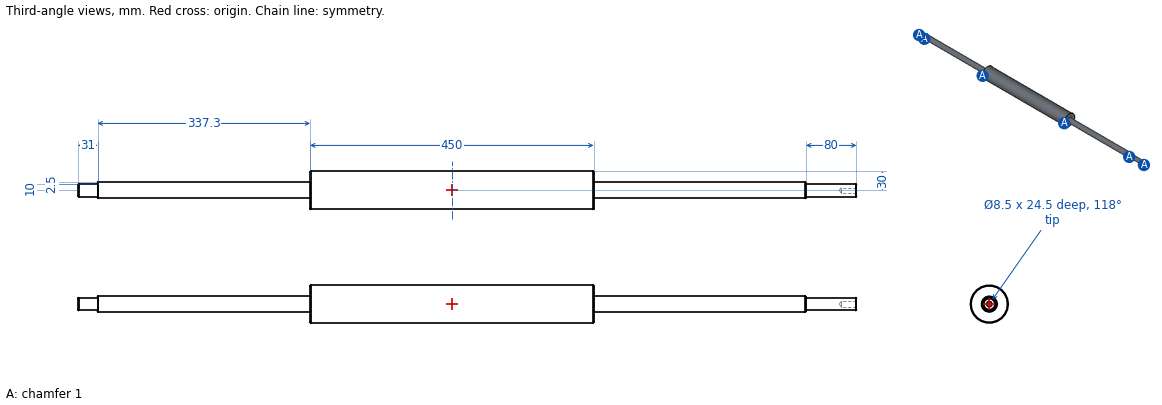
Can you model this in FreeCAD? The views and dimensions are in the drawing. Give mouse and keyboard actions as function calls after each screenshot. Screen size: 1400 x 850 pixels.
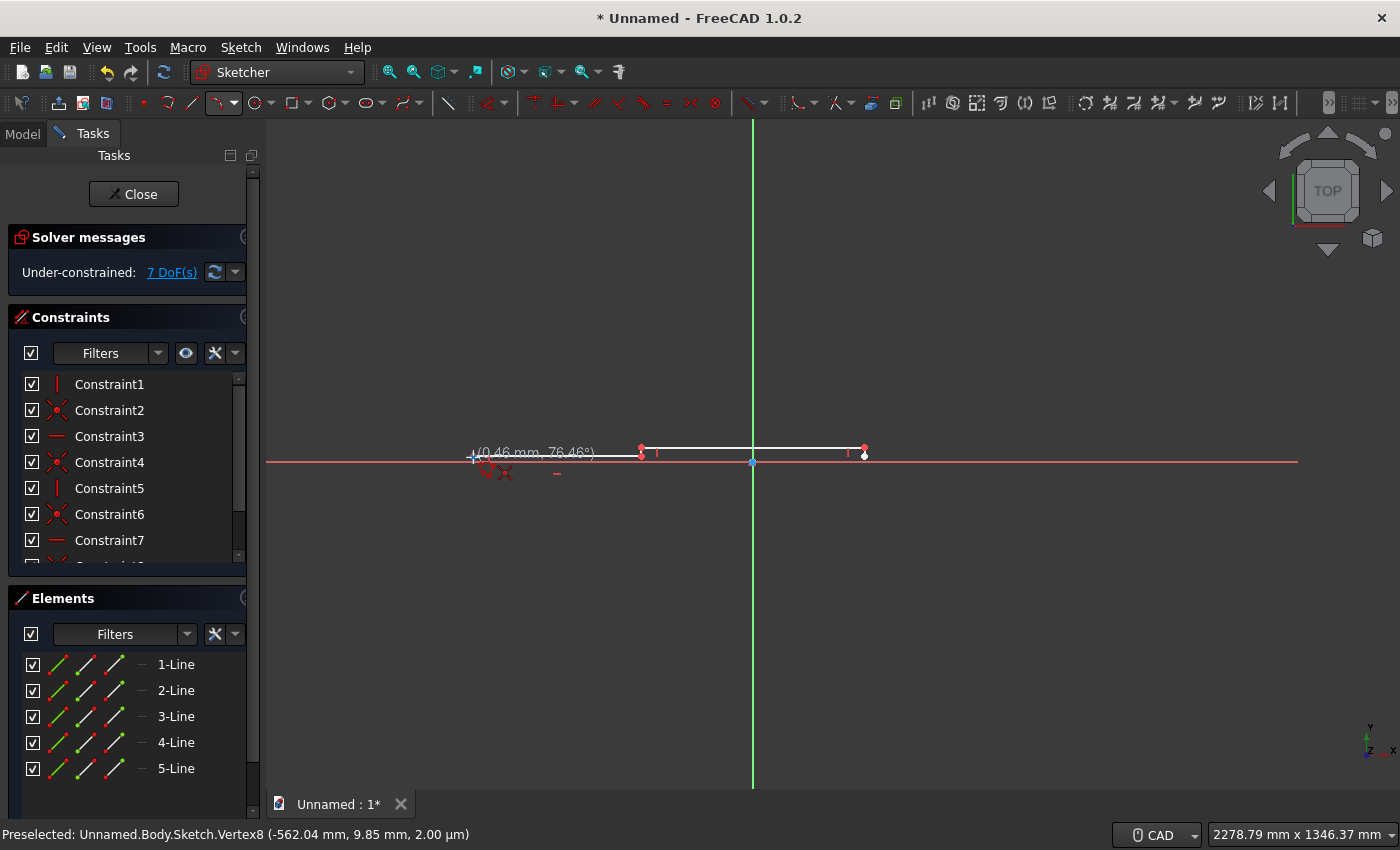
scroll(458, 457, up, 6)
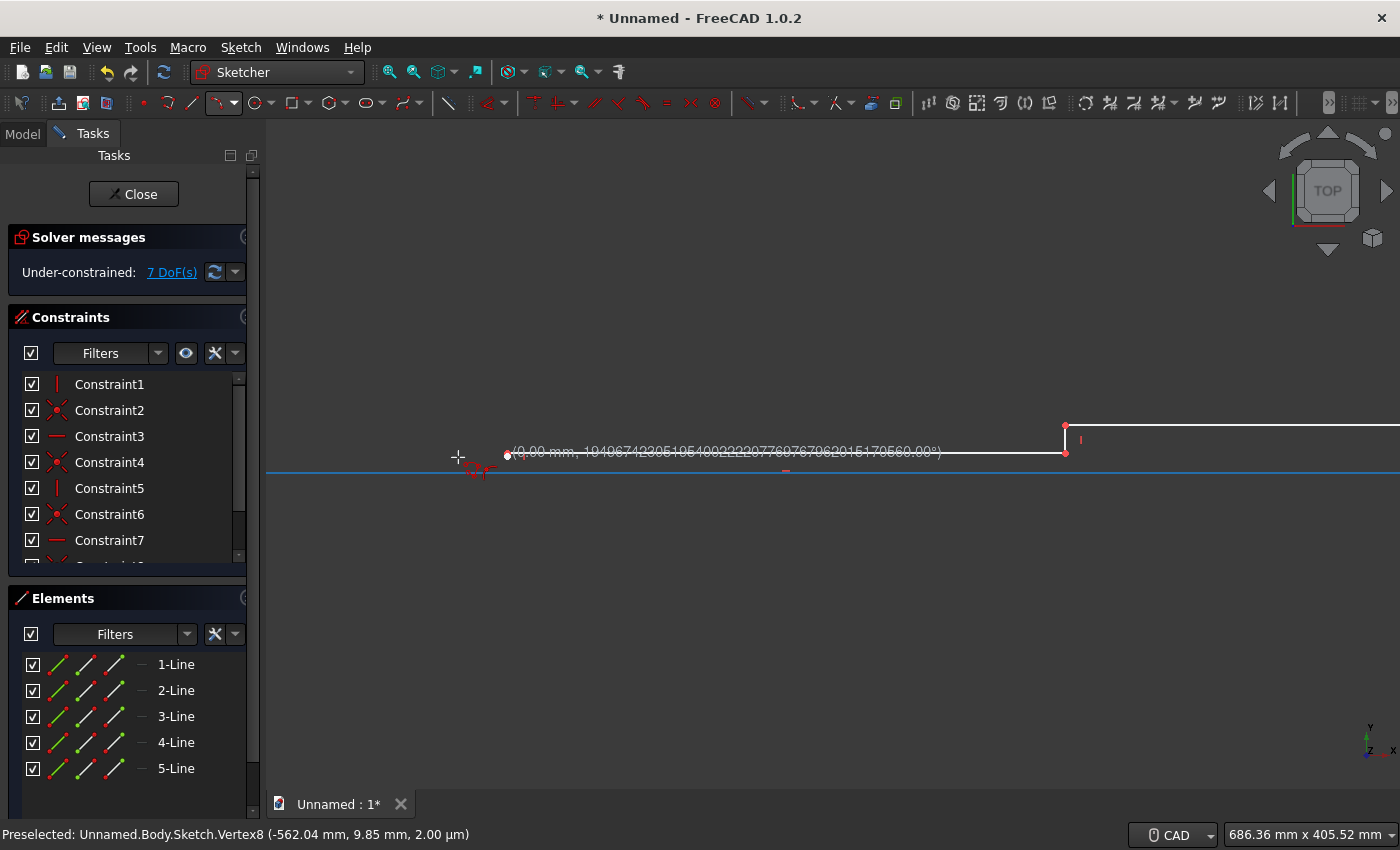
click(456, 457)
click(456, 473)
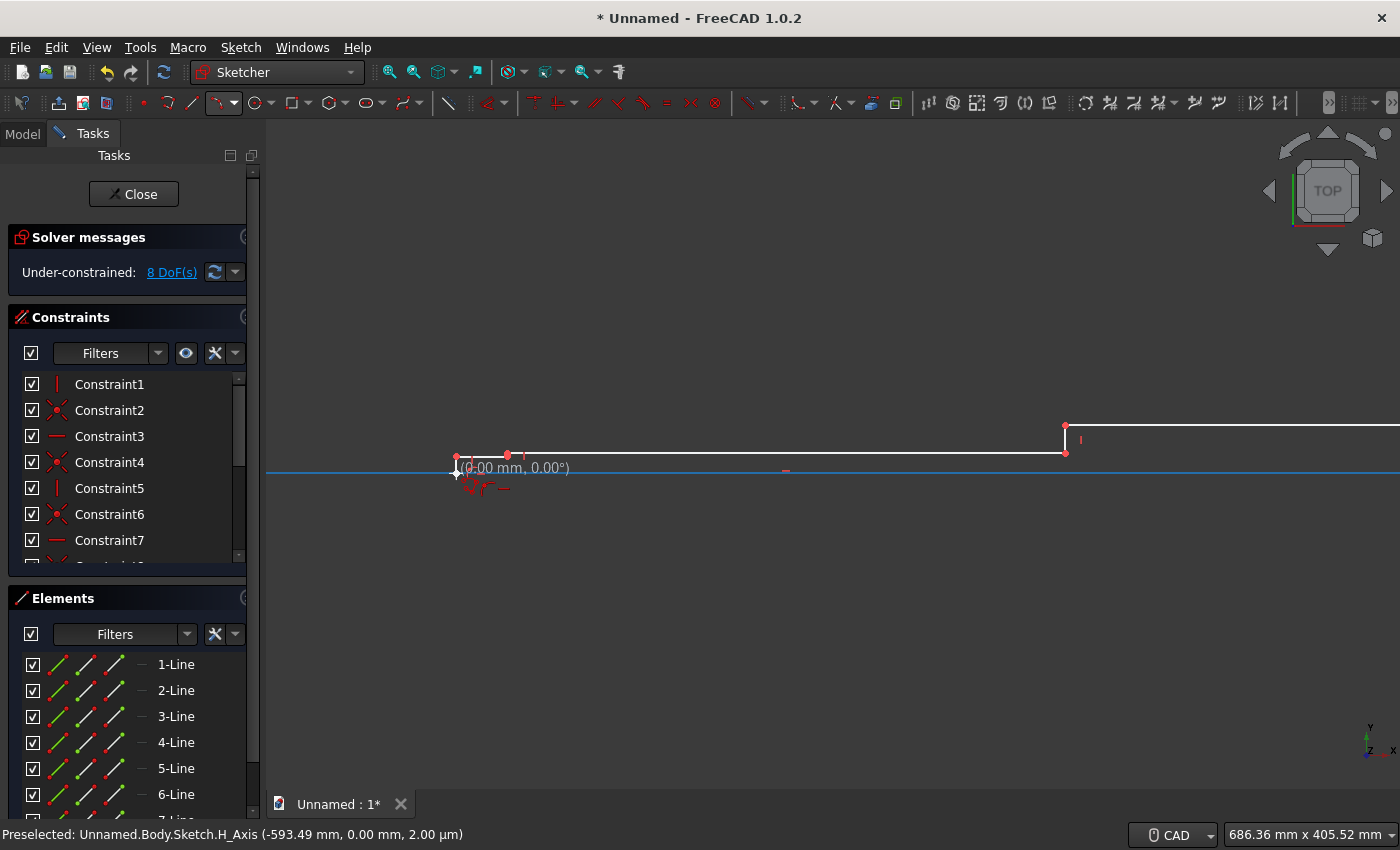
scroll(457, 456, down, 6)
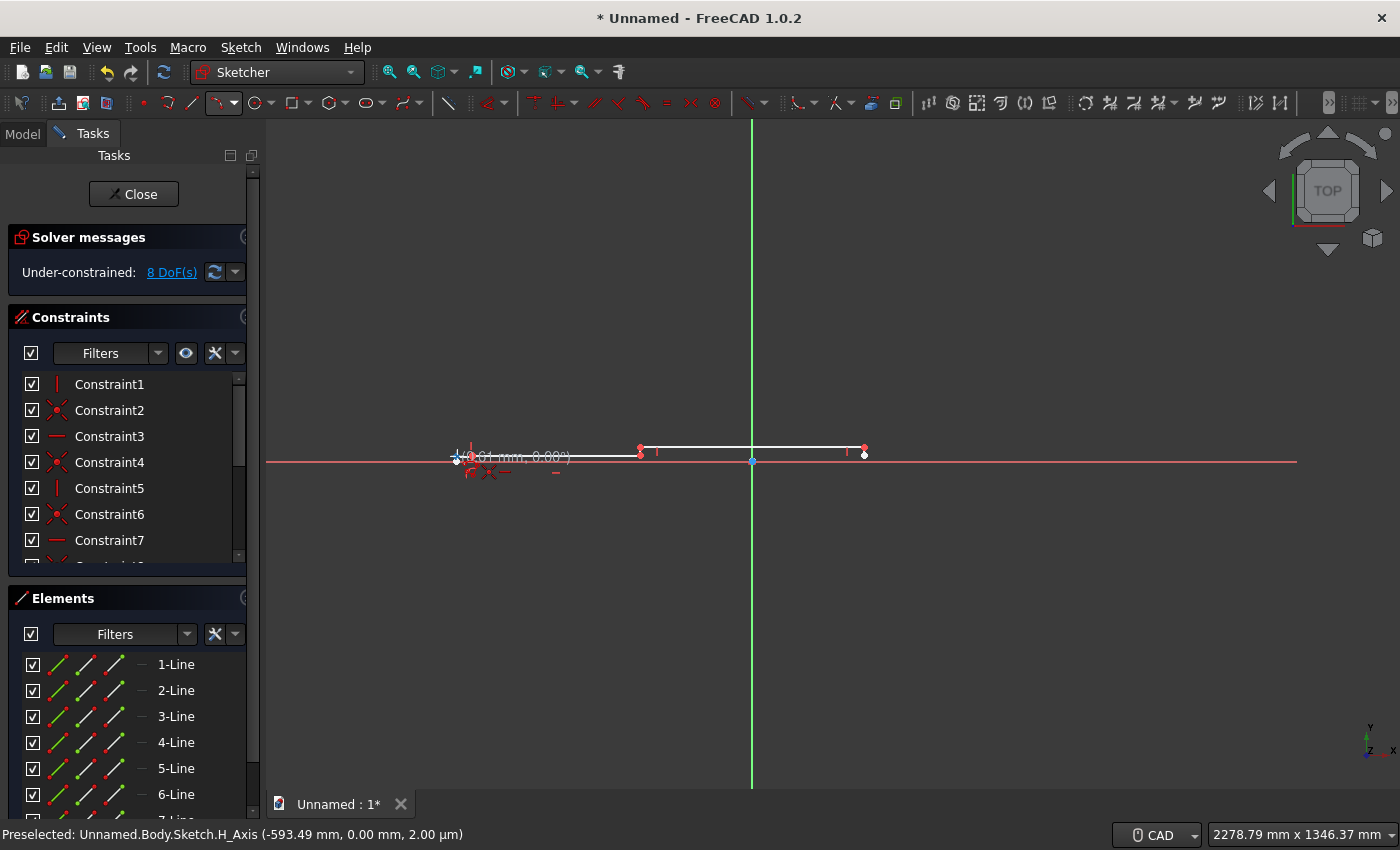
click(1072, 453)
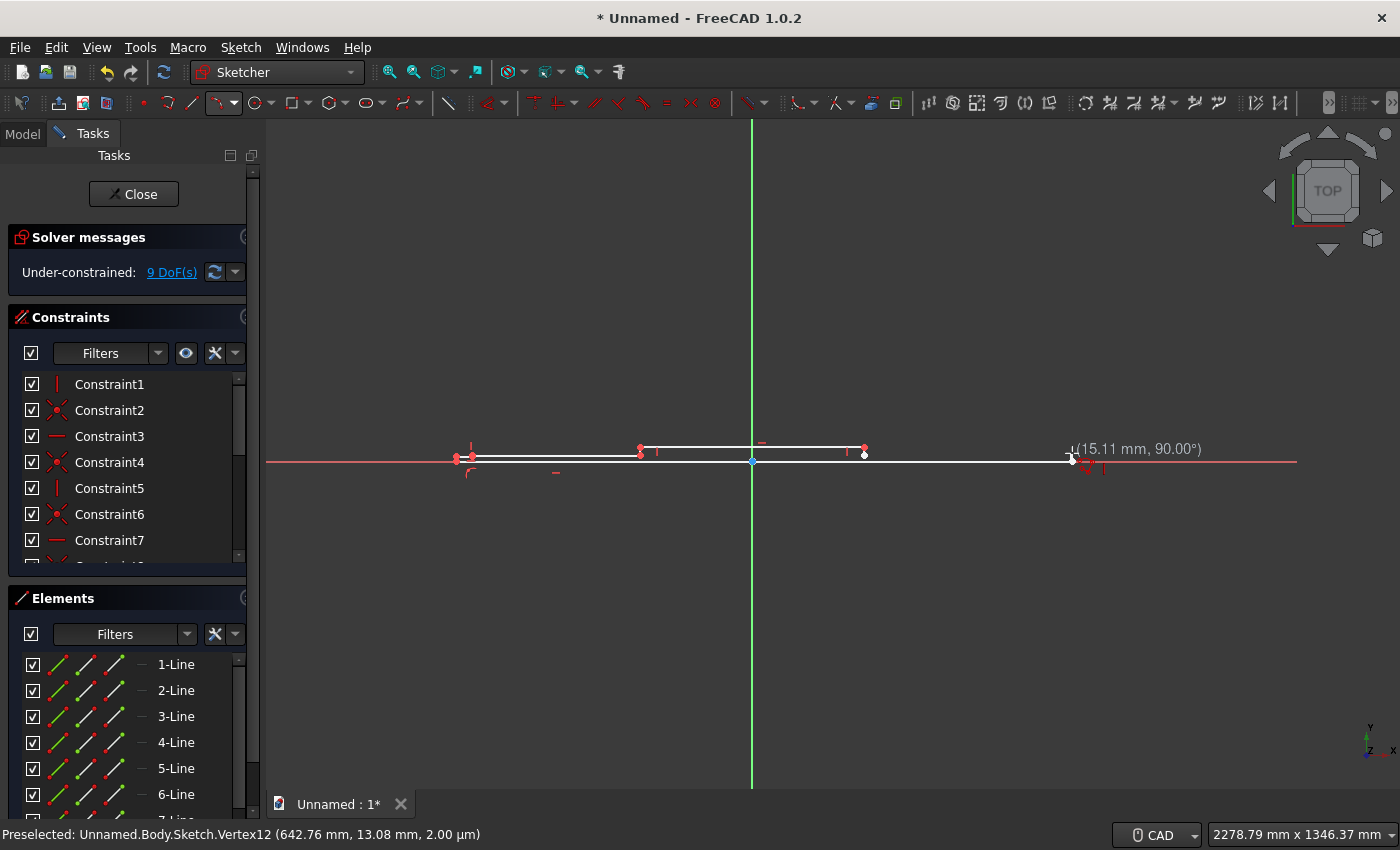
scroll(1072, 457, up, 6)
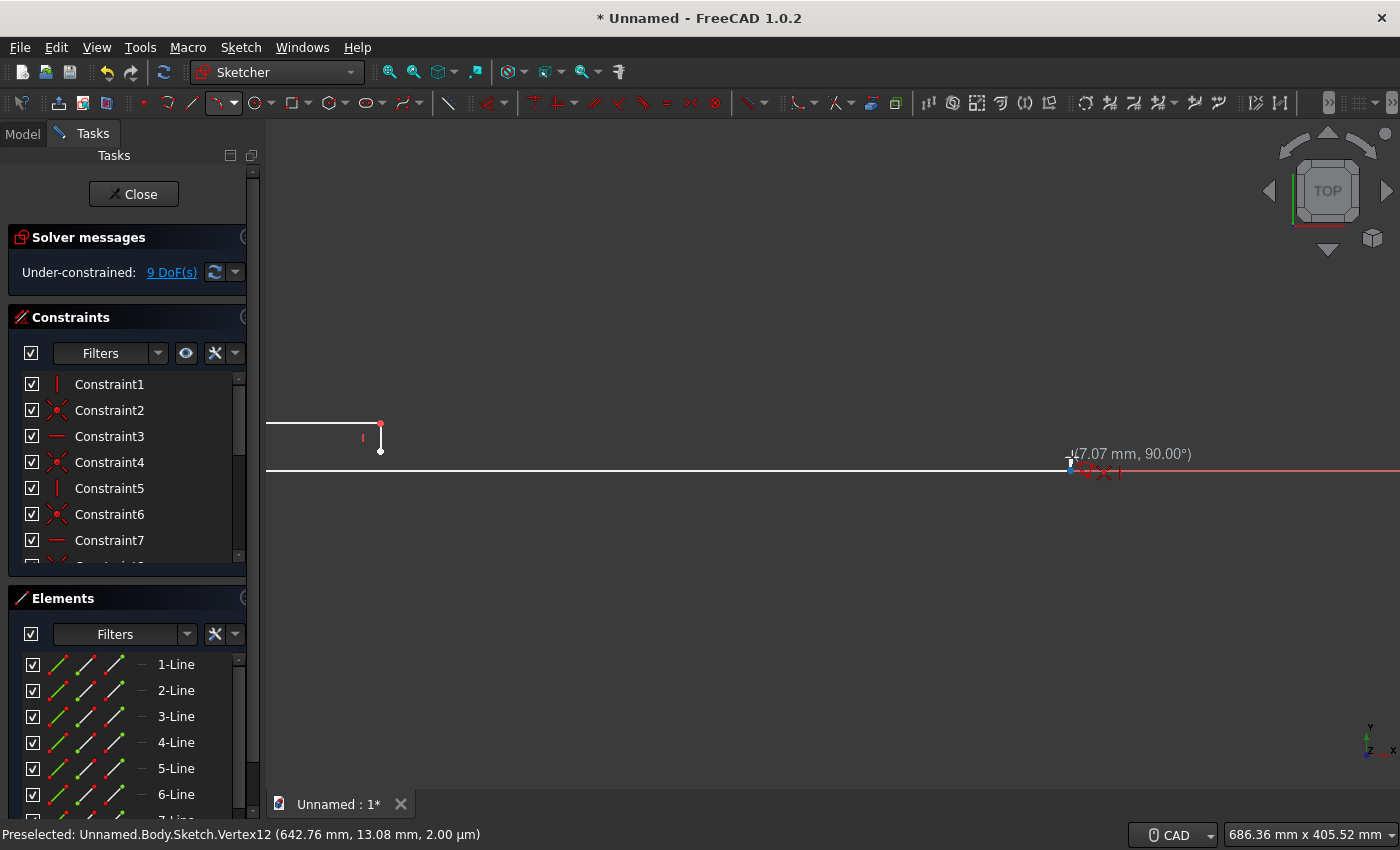
click(1070, 454)
click(937, 454)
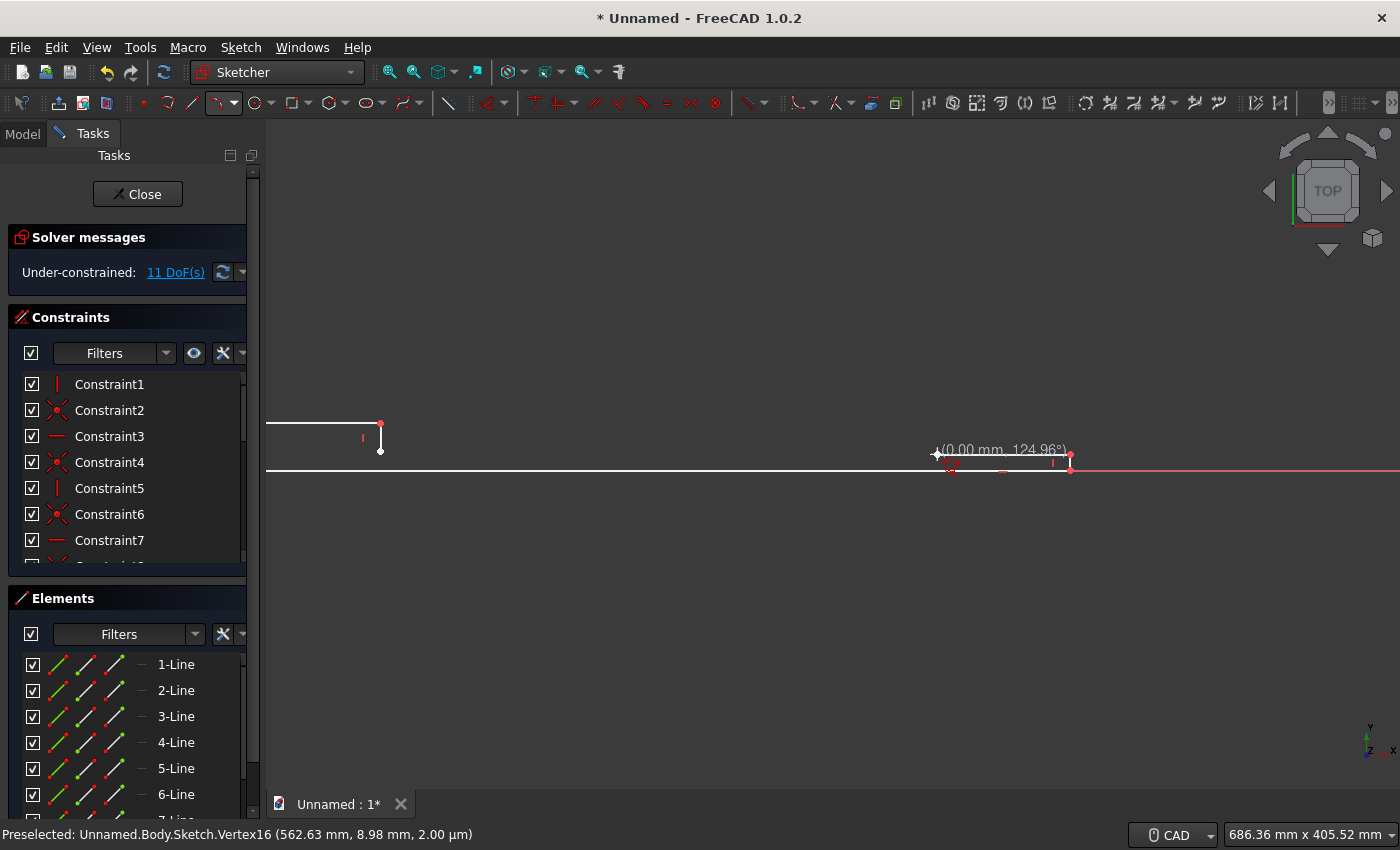
scroll(937, 450, up, 7)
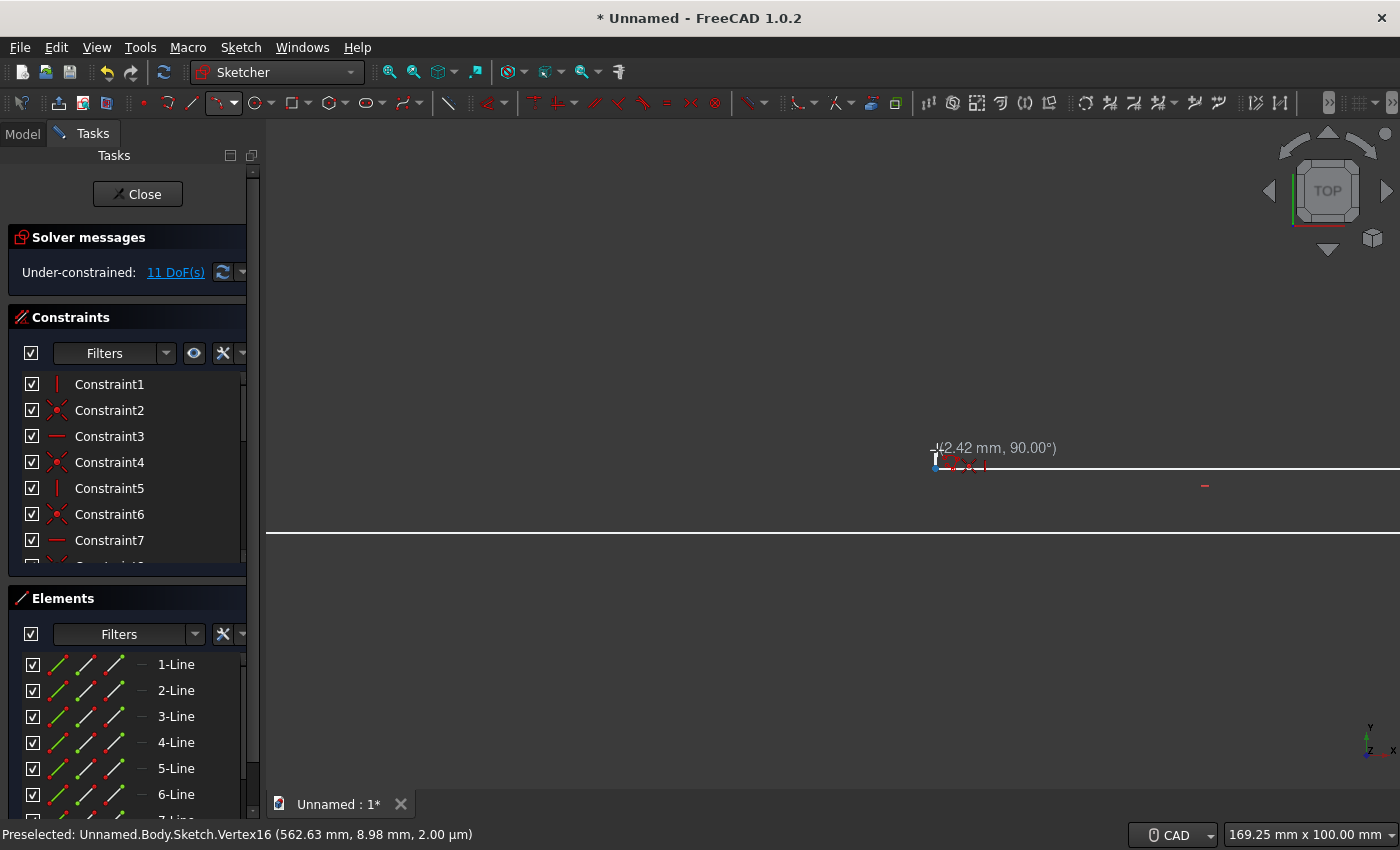
click(935, 449)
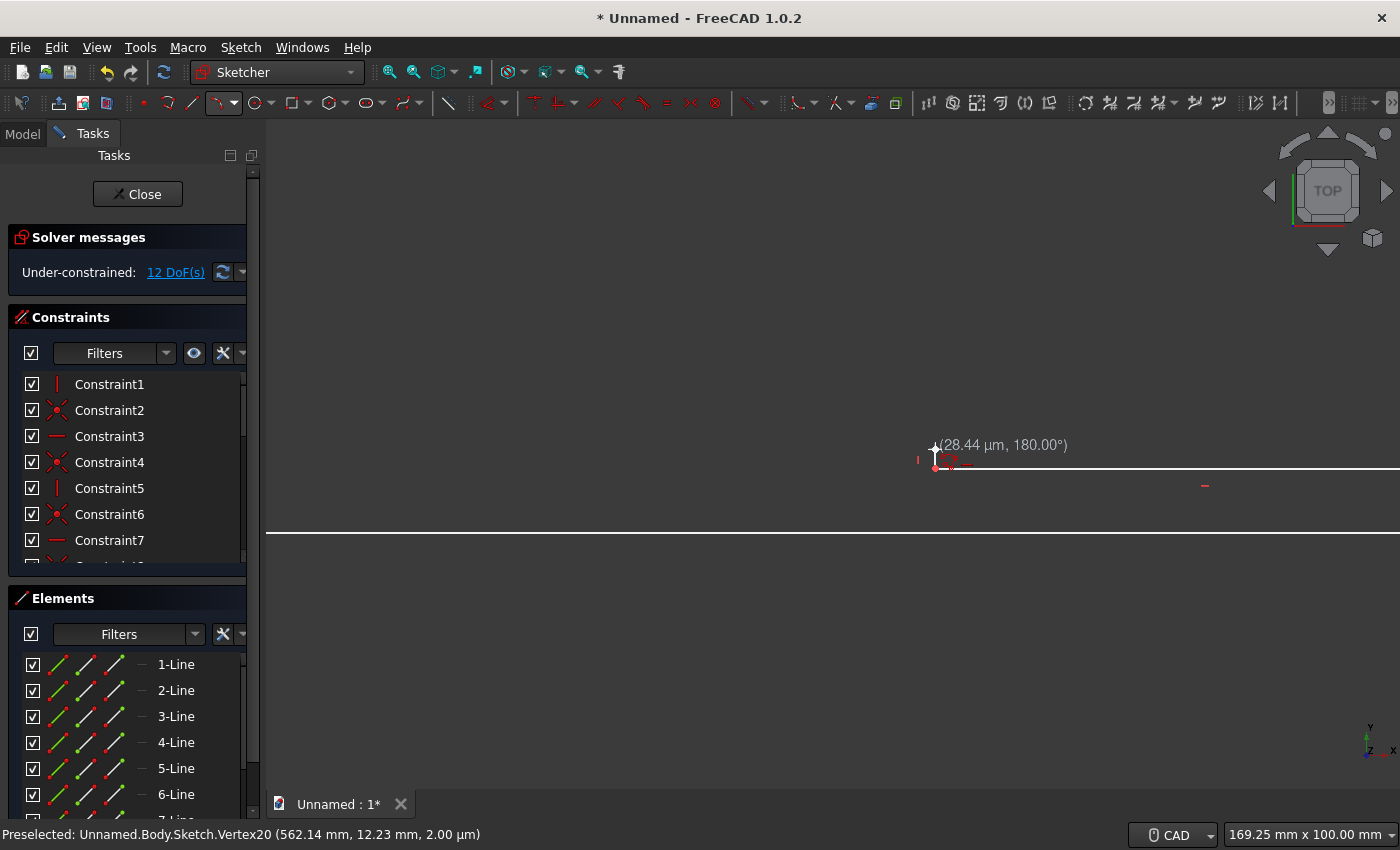
scroll(1040, 456, down, 13)